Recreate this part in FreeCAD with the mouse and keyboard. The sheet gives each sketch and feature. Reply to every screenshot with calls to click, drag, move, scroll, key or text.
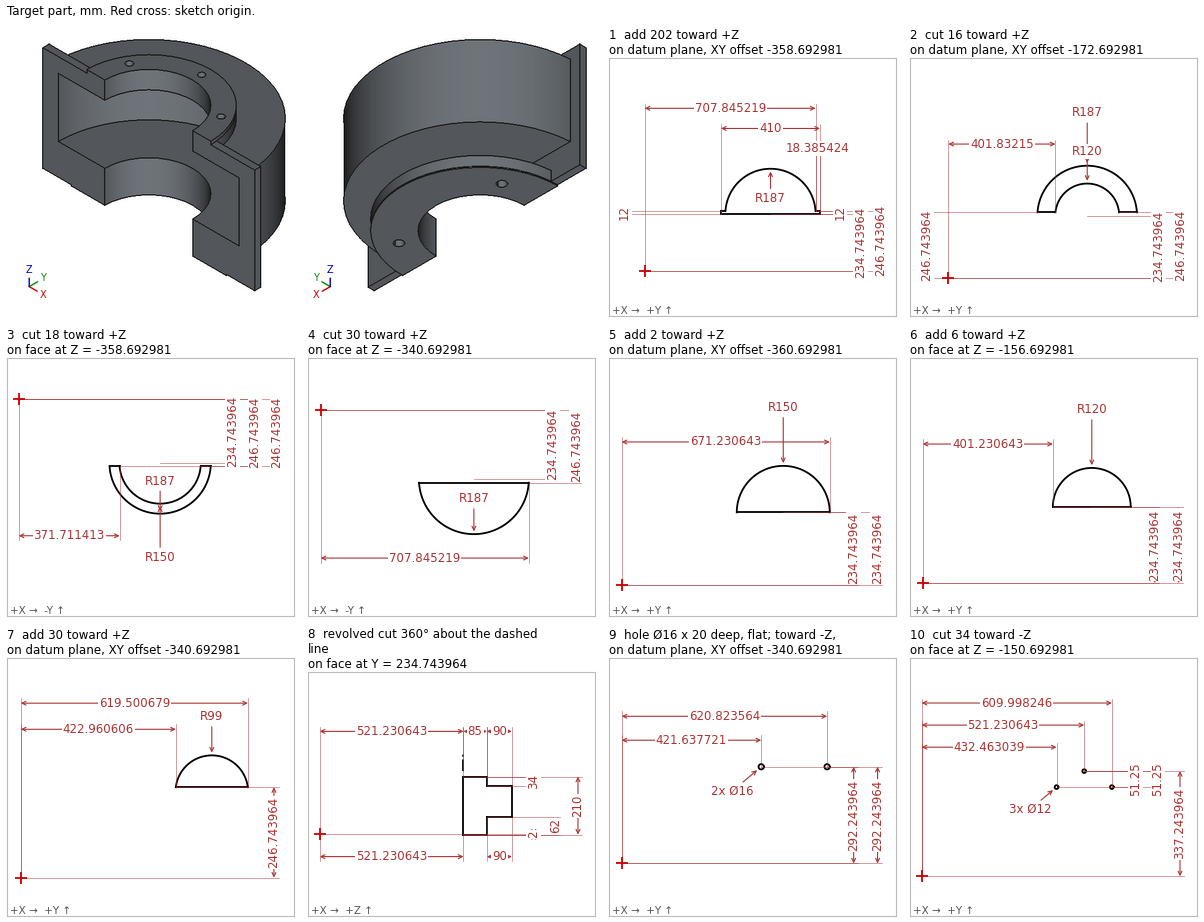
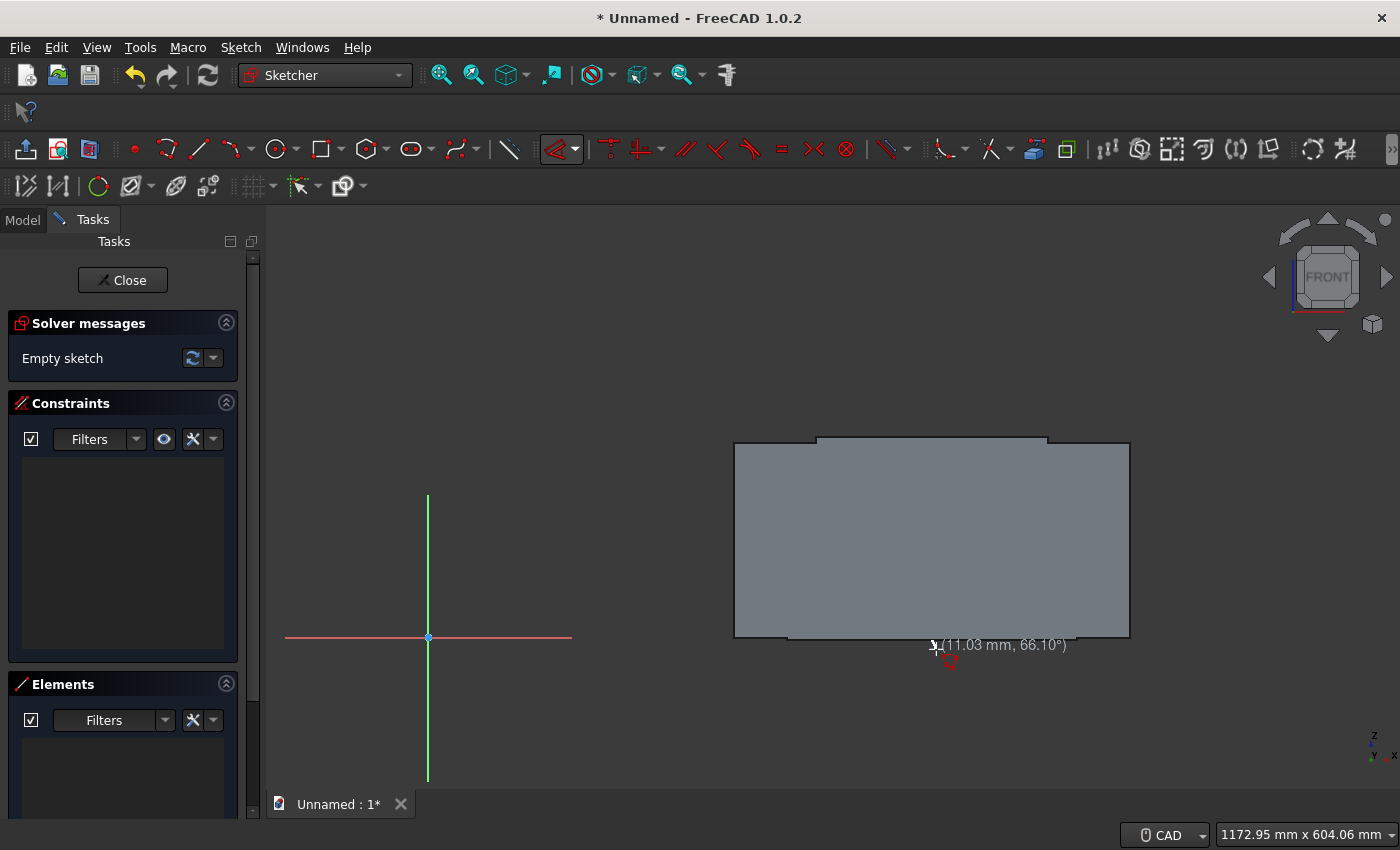
click(932, 437)
click(1014, 437)
click(1014, 470)
click(1101, 470)
click(1101, 580)
click(1014, 580)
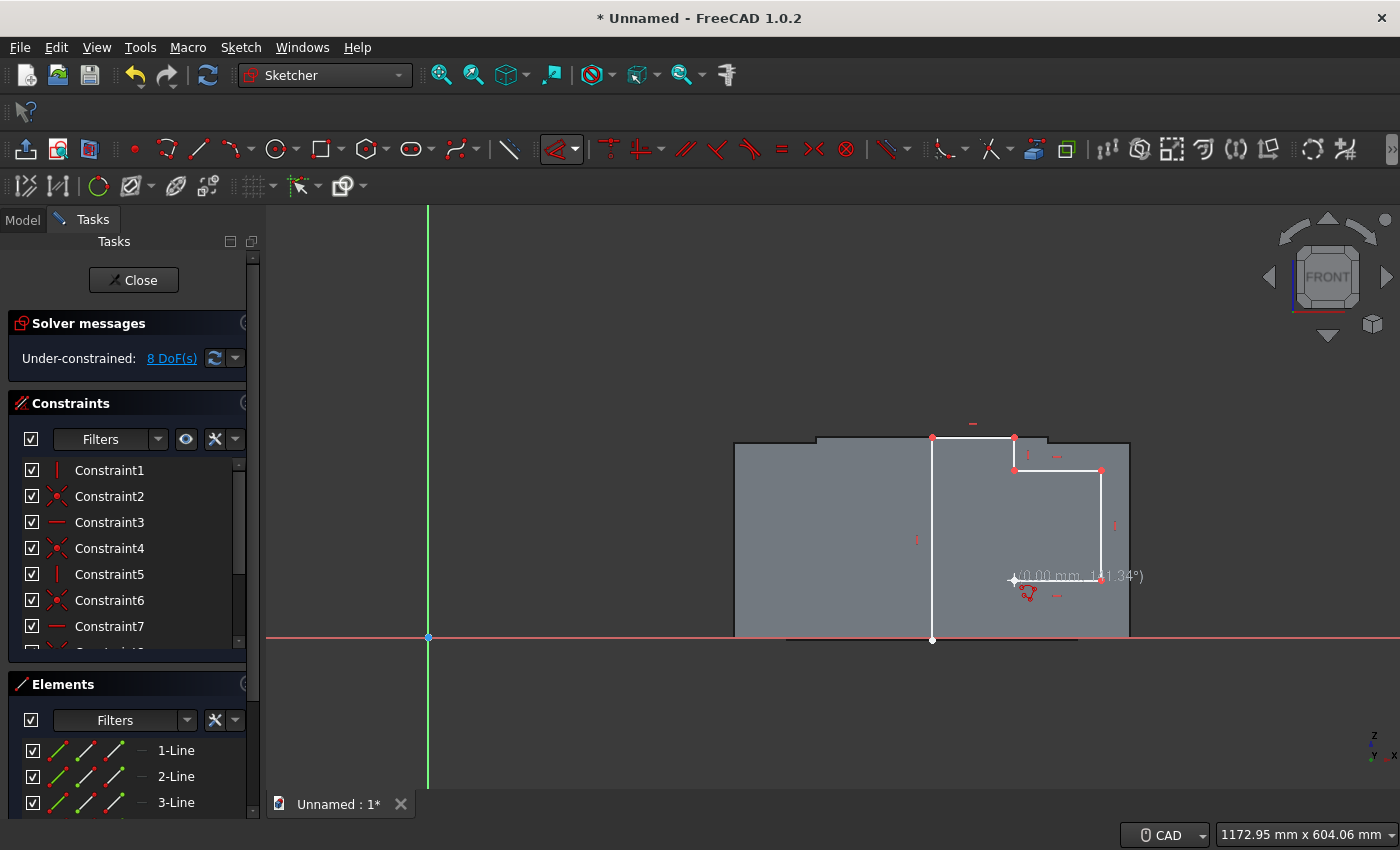
scroll(1014, 640, up, 11)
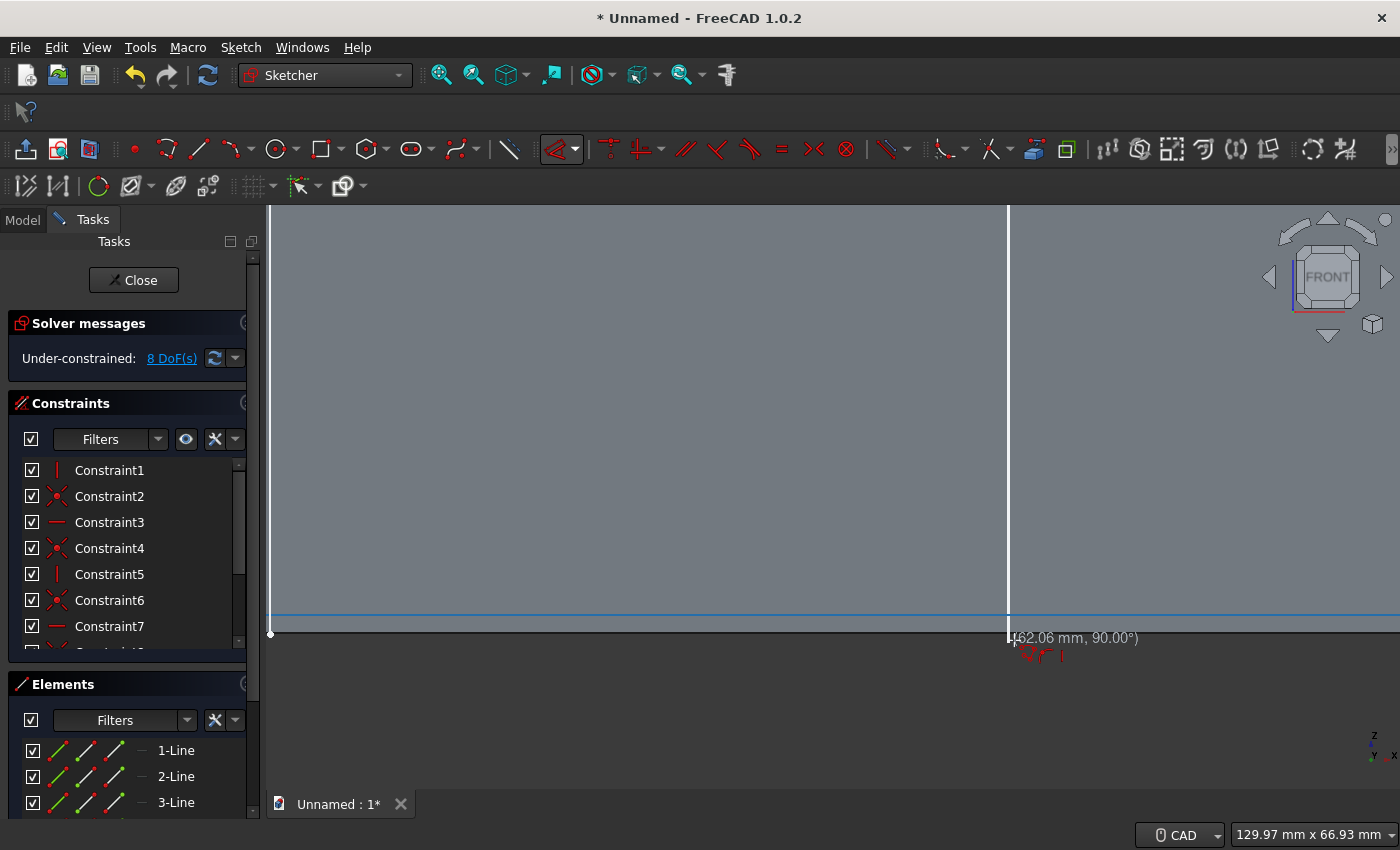
click(1009, 633)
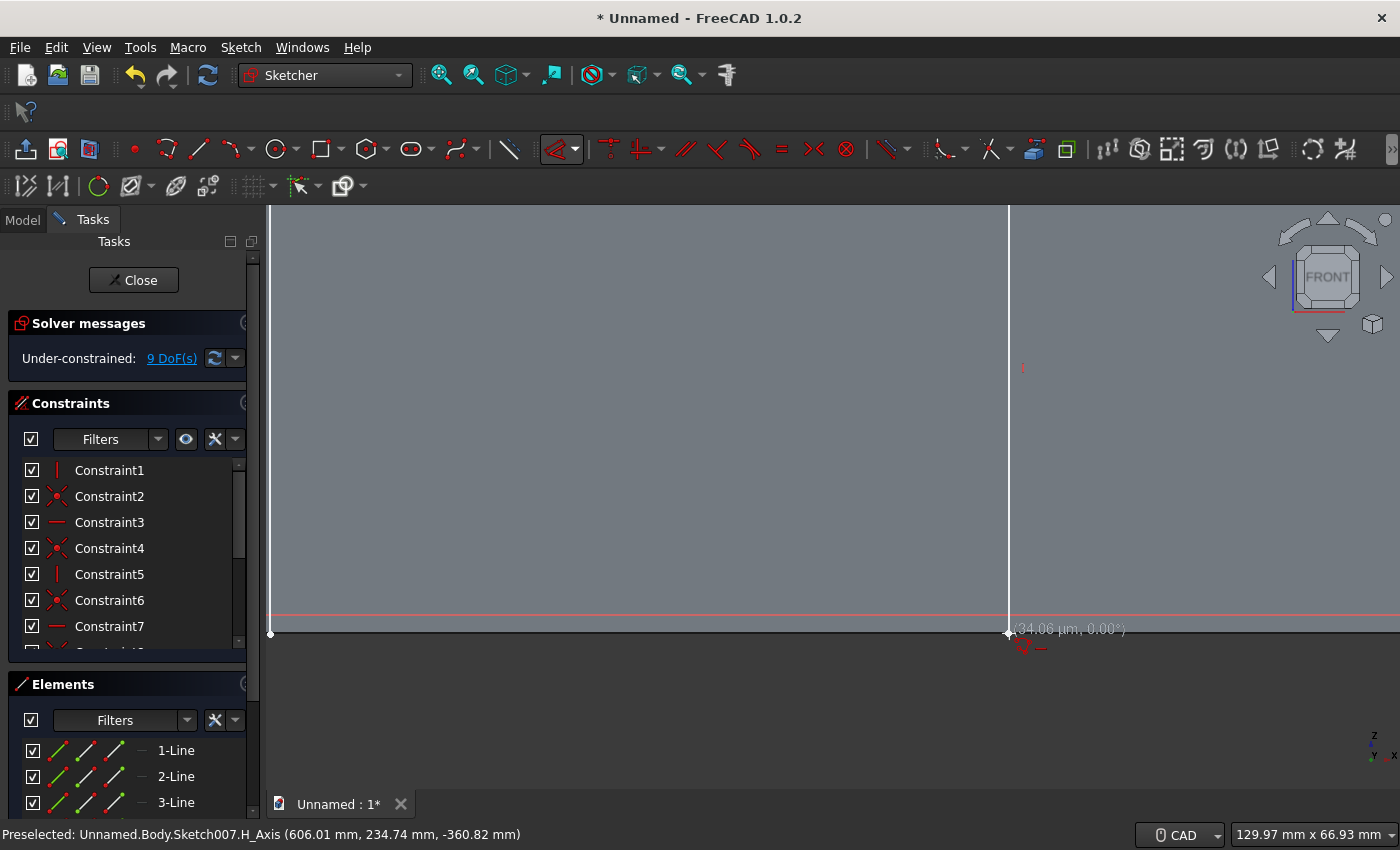
scroll(1014, 640, down, 11)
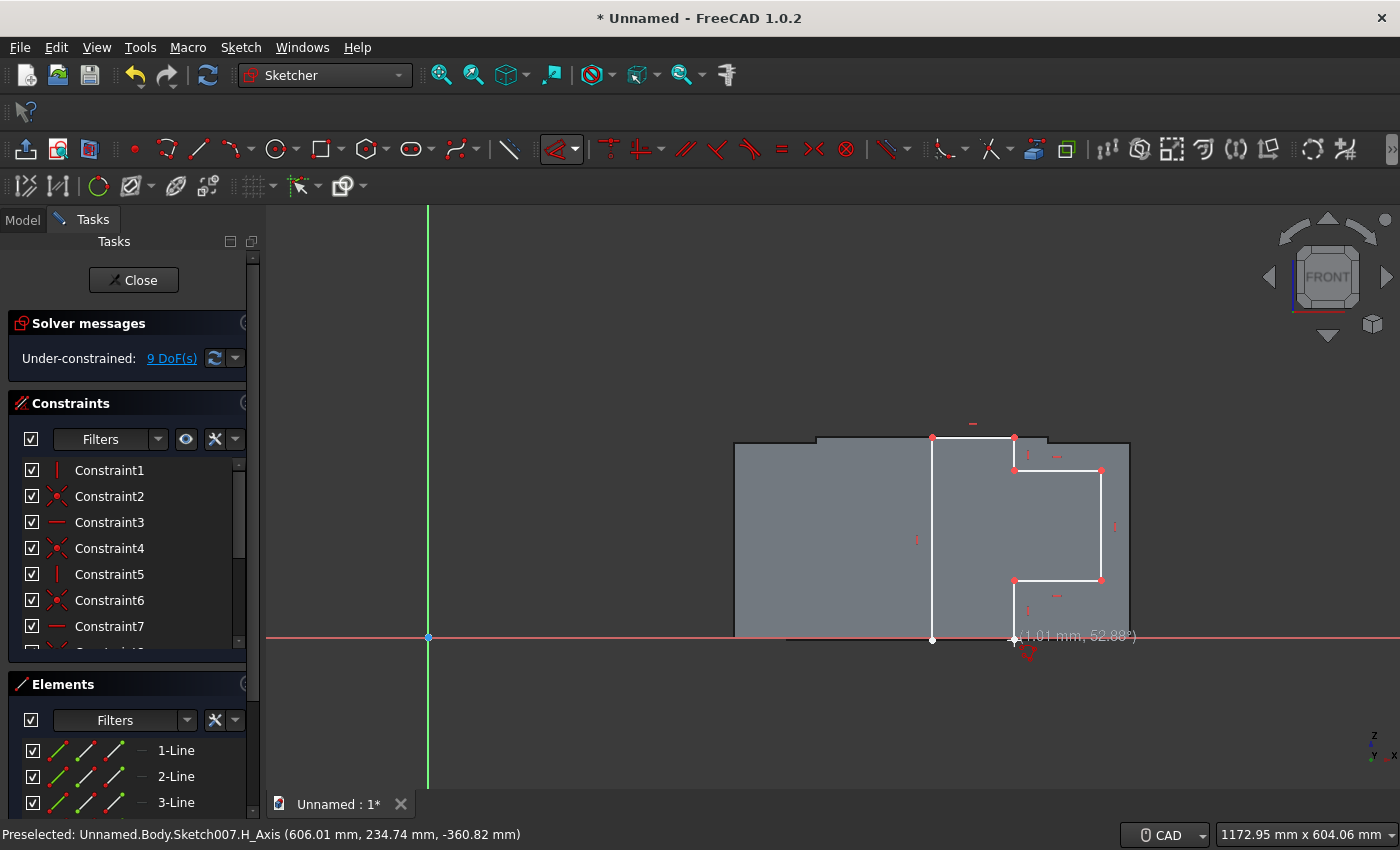
scroll(932, 640, up, 11)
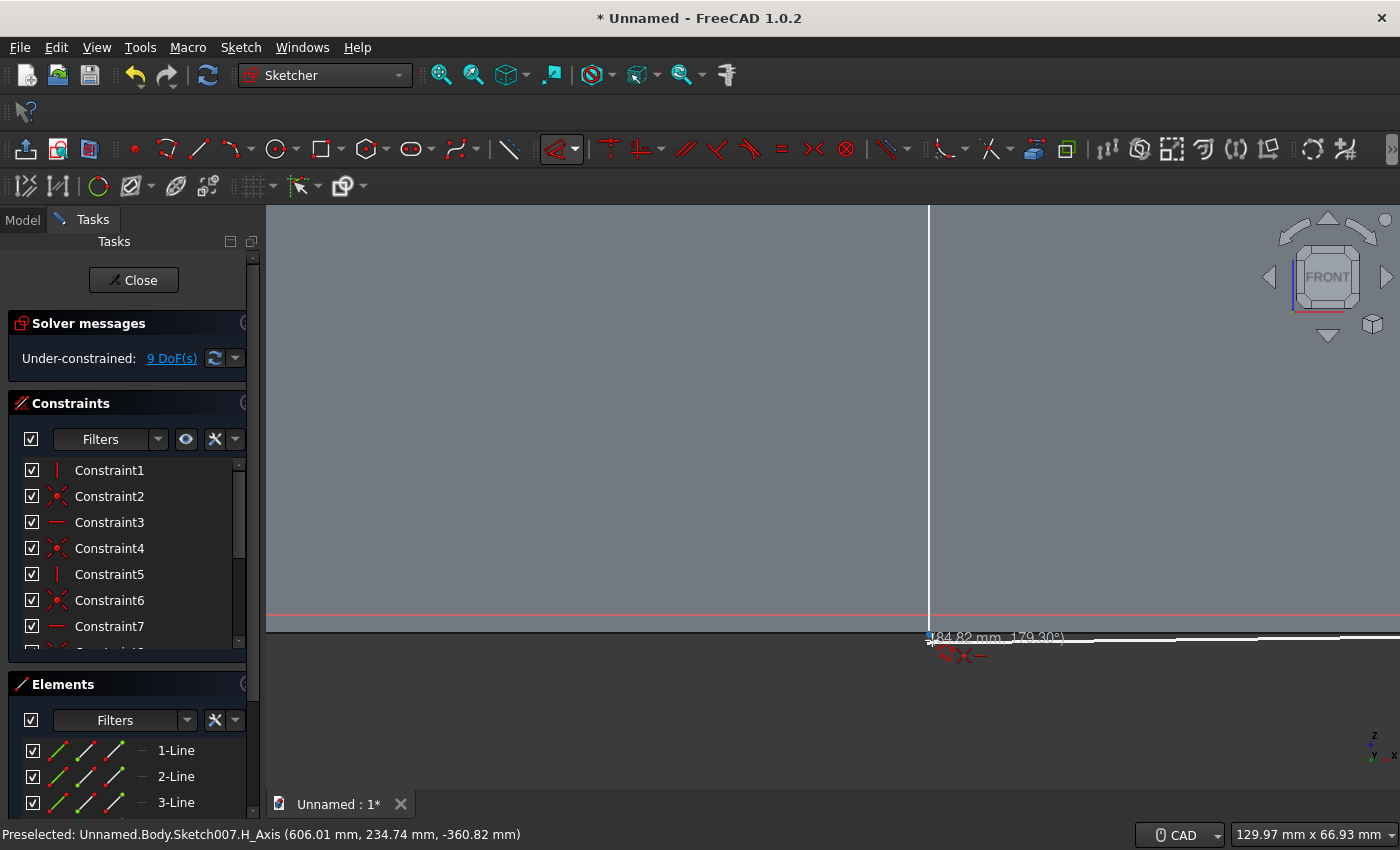
click(929, 634)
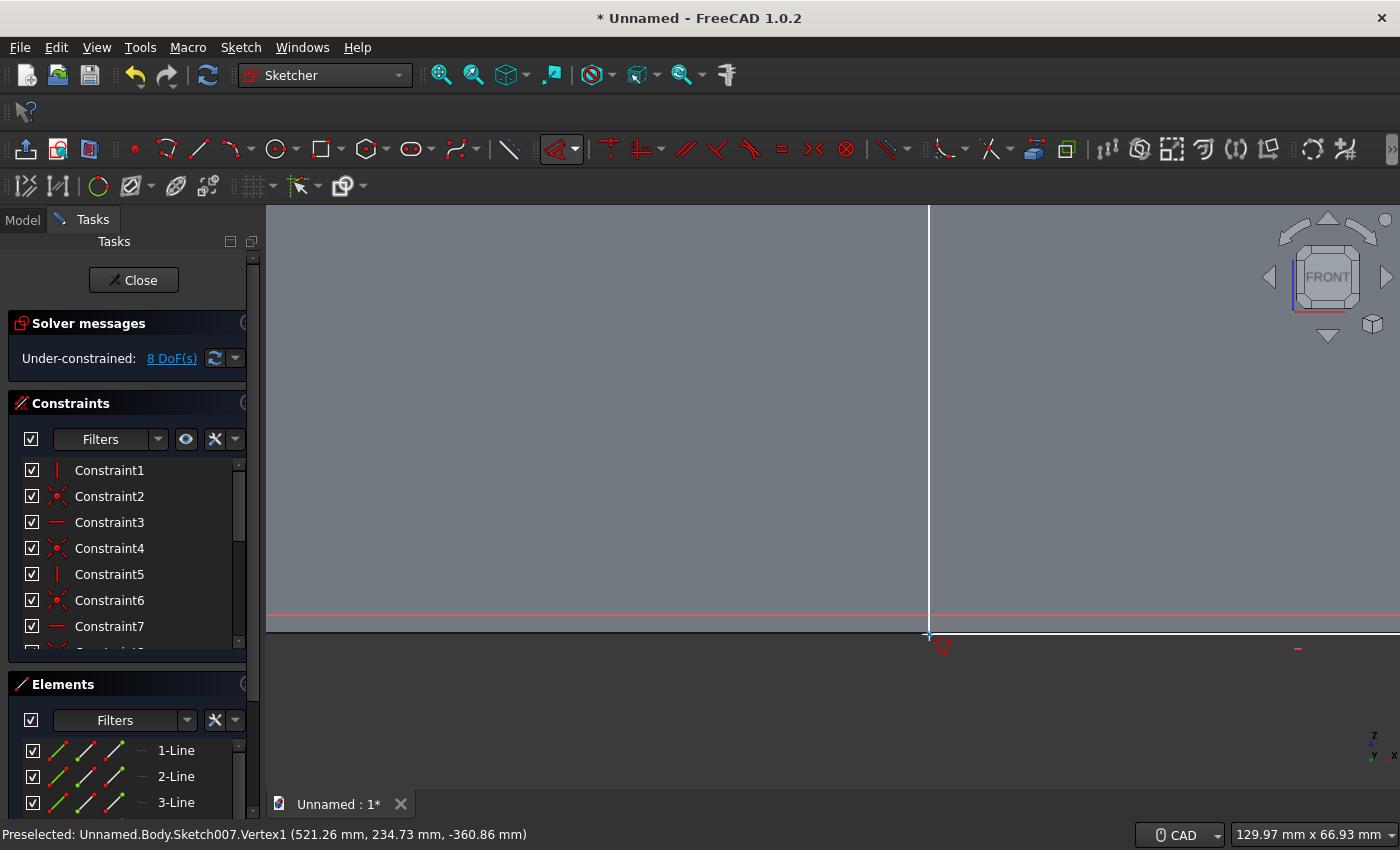
key(g)
key(l)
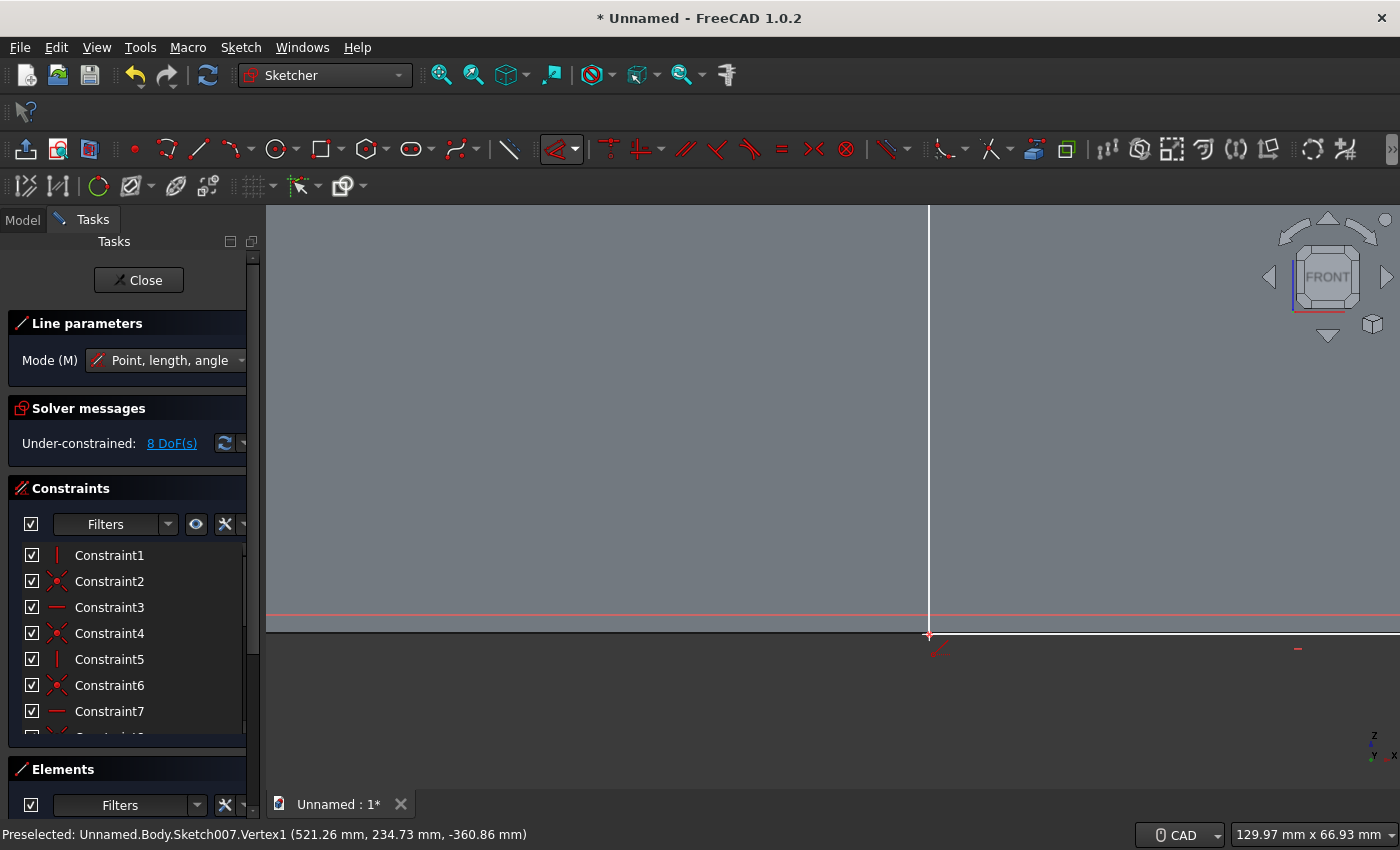
scroll(932, 640, down, 11)